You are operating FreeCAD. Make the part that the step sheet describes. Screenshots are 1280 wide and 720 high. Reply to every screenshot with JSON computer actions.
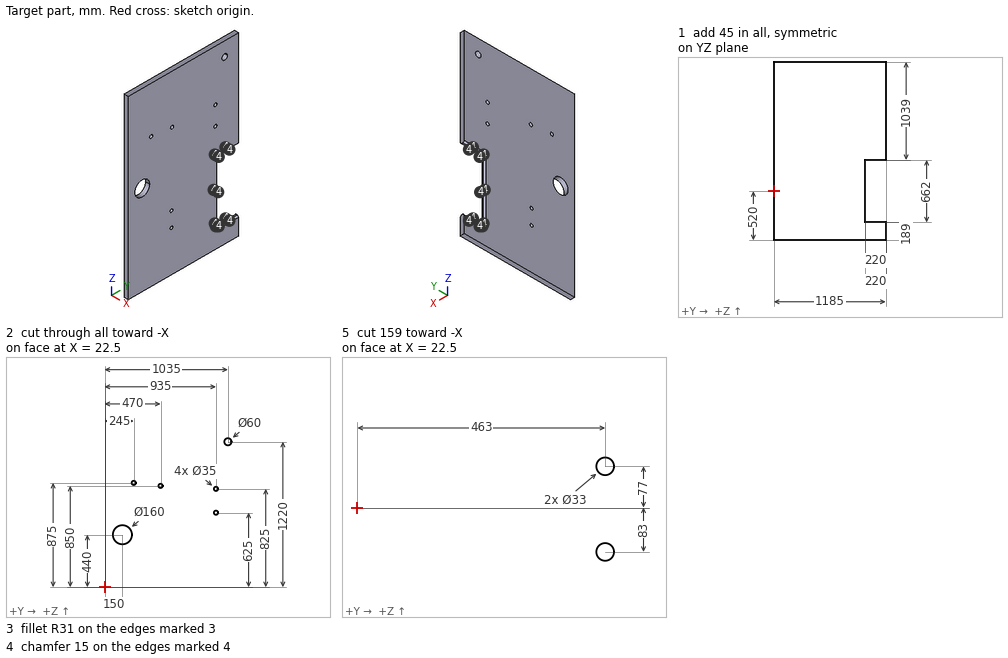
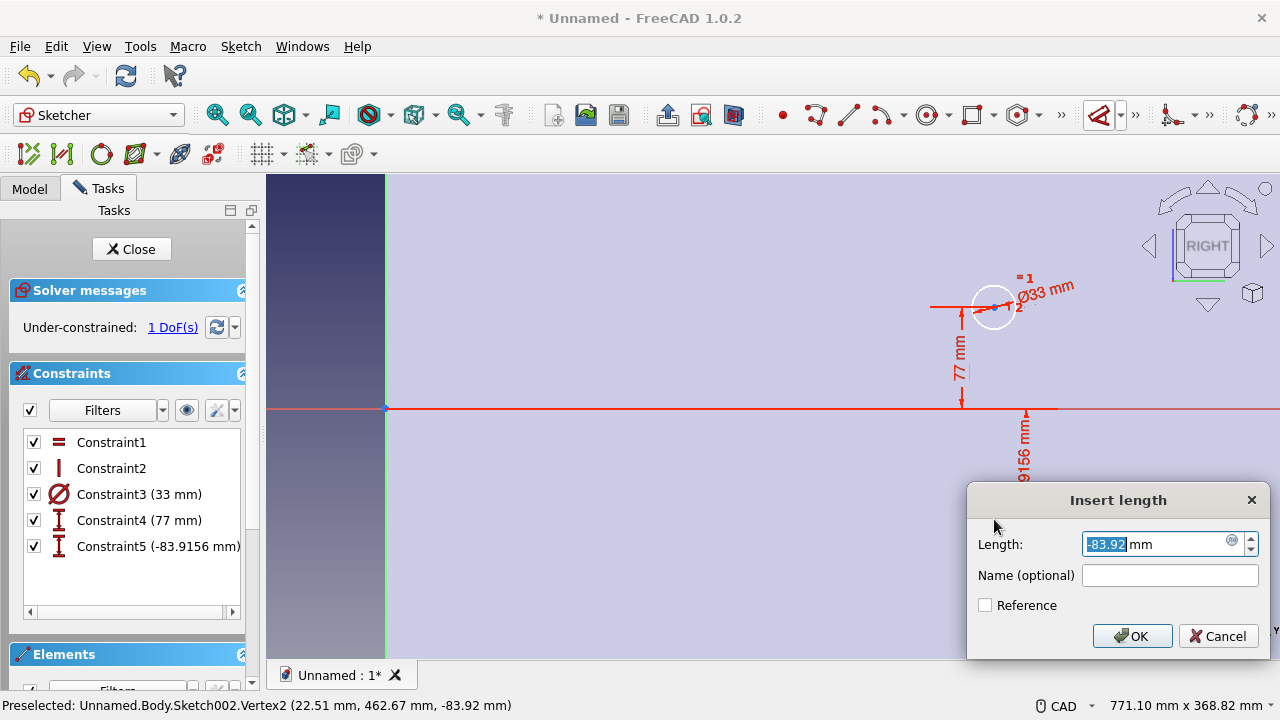
{"action": "type", "text": "-83"}
{"action": "key", "text": "Return"}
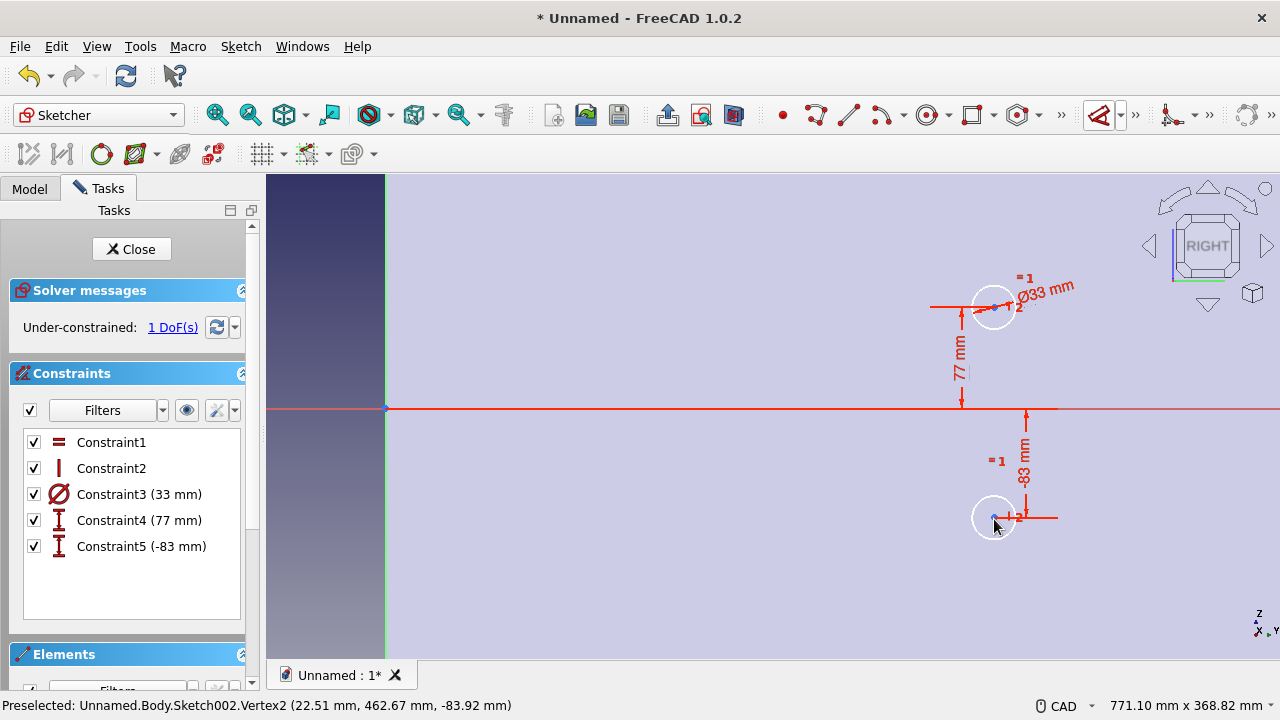
{"action": "left_click", "coordinate": [994, 307]}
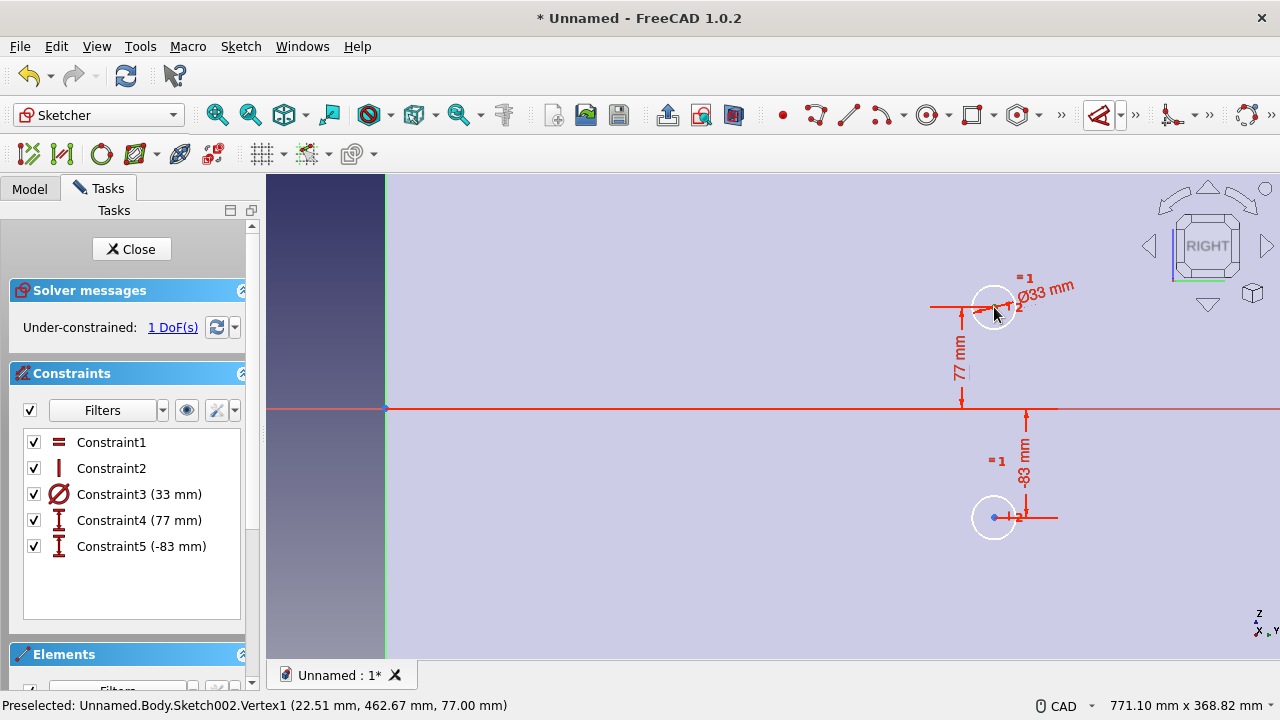
{"action": "left_click", "coordinate": [1120, 116]}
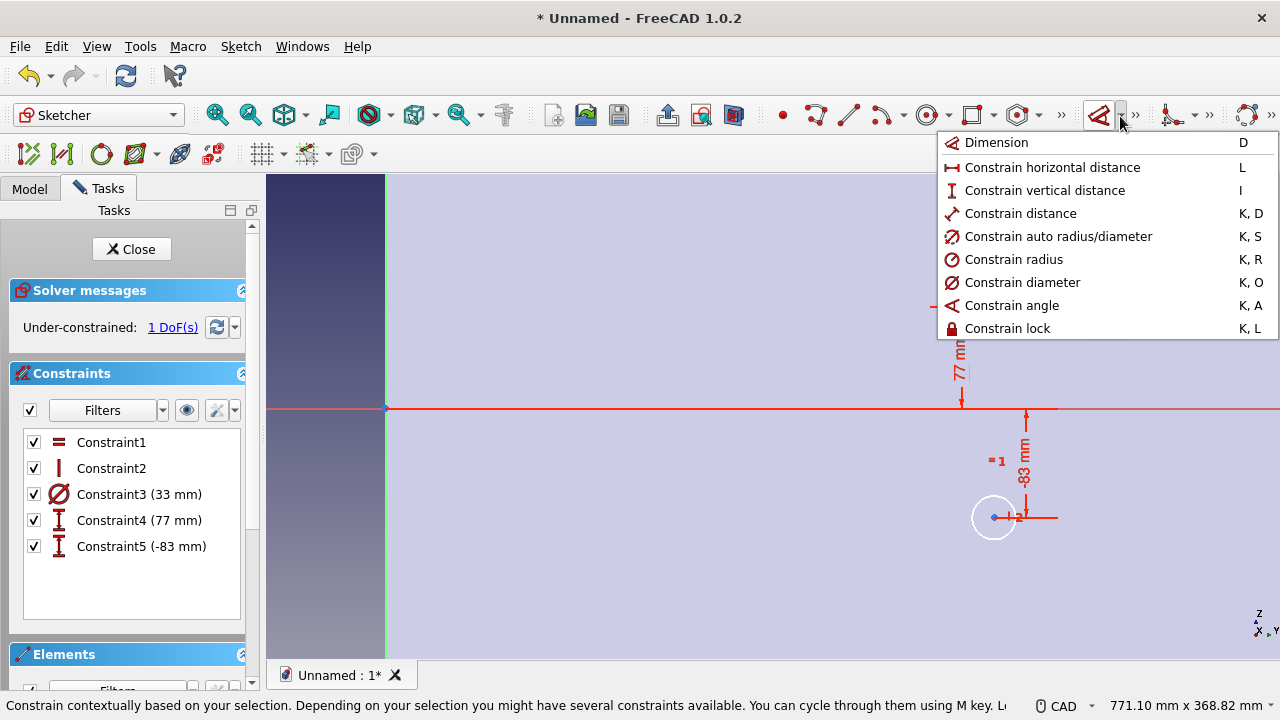
{"action": "left_click", "coordinate": [1108, 168]}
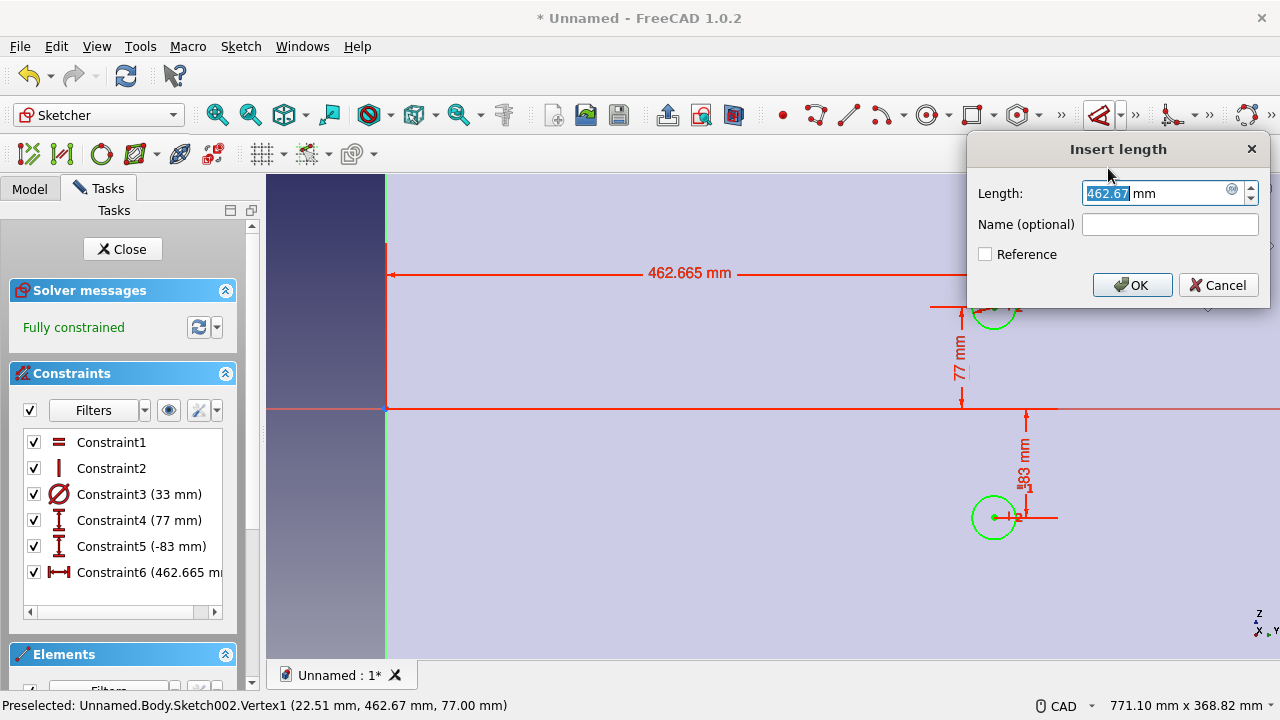
{"action": "type", "text": "463"}
{"action": "key", "text": "Return"}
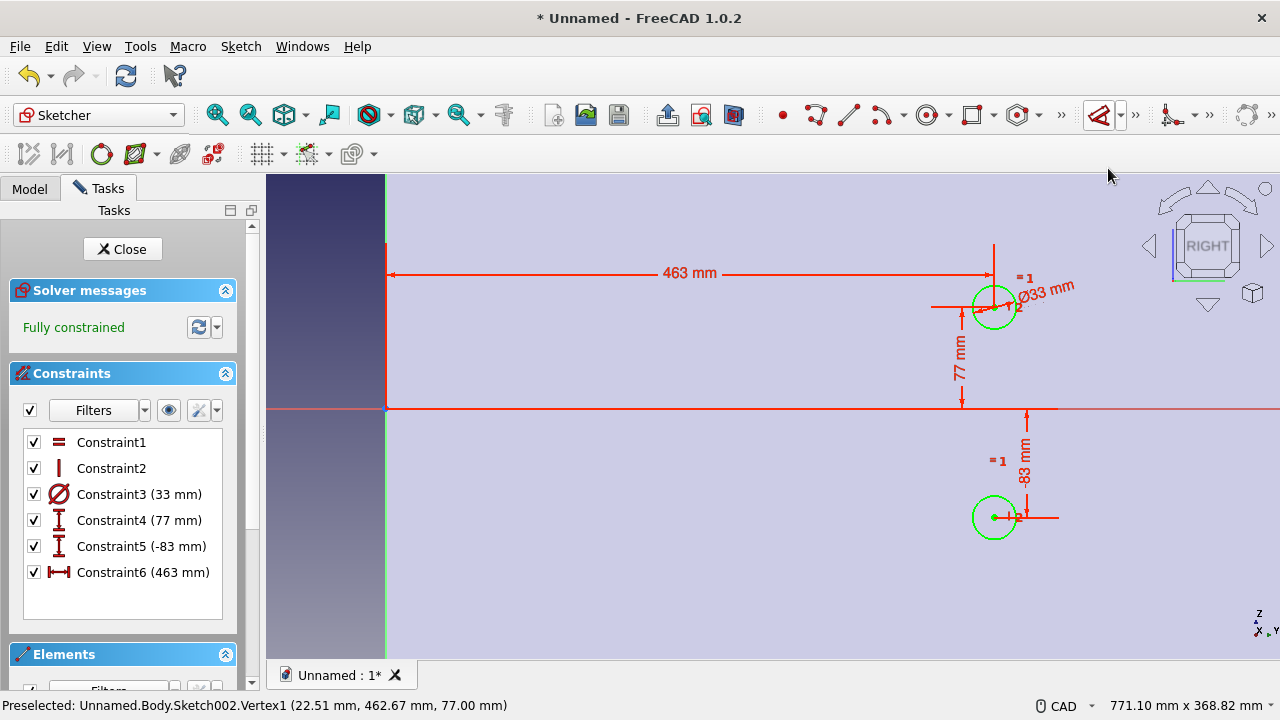
{"action": "left_click", "coordinate": [123, 249]}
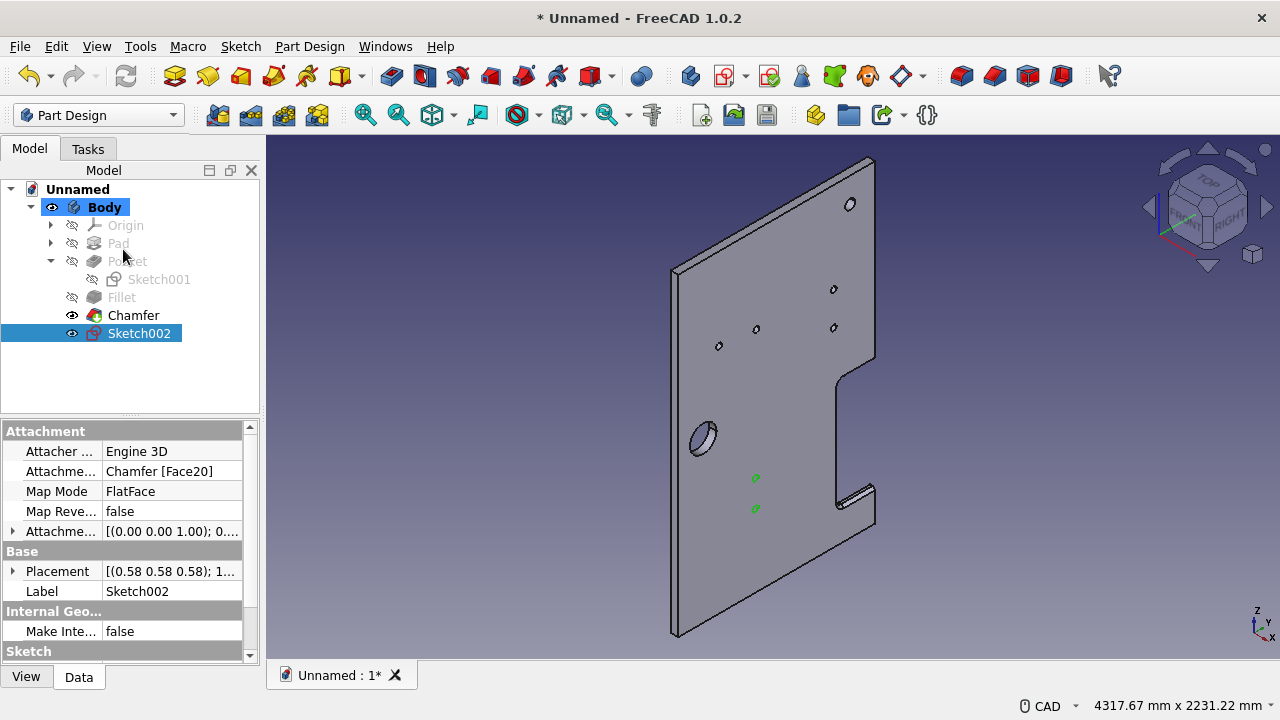
{"action": "left_click", "coordinate": [392, 76]}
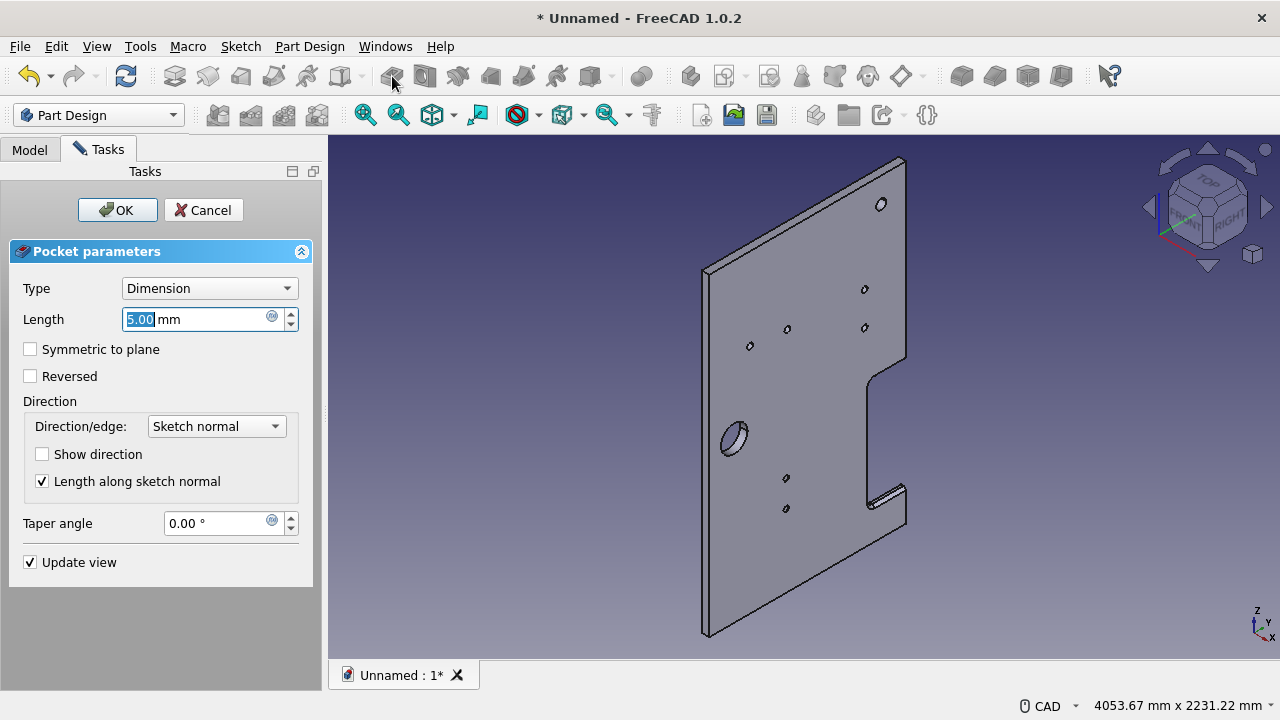
{"action": "type", "text": "159"}
{"action": "key", "text": "Tab"}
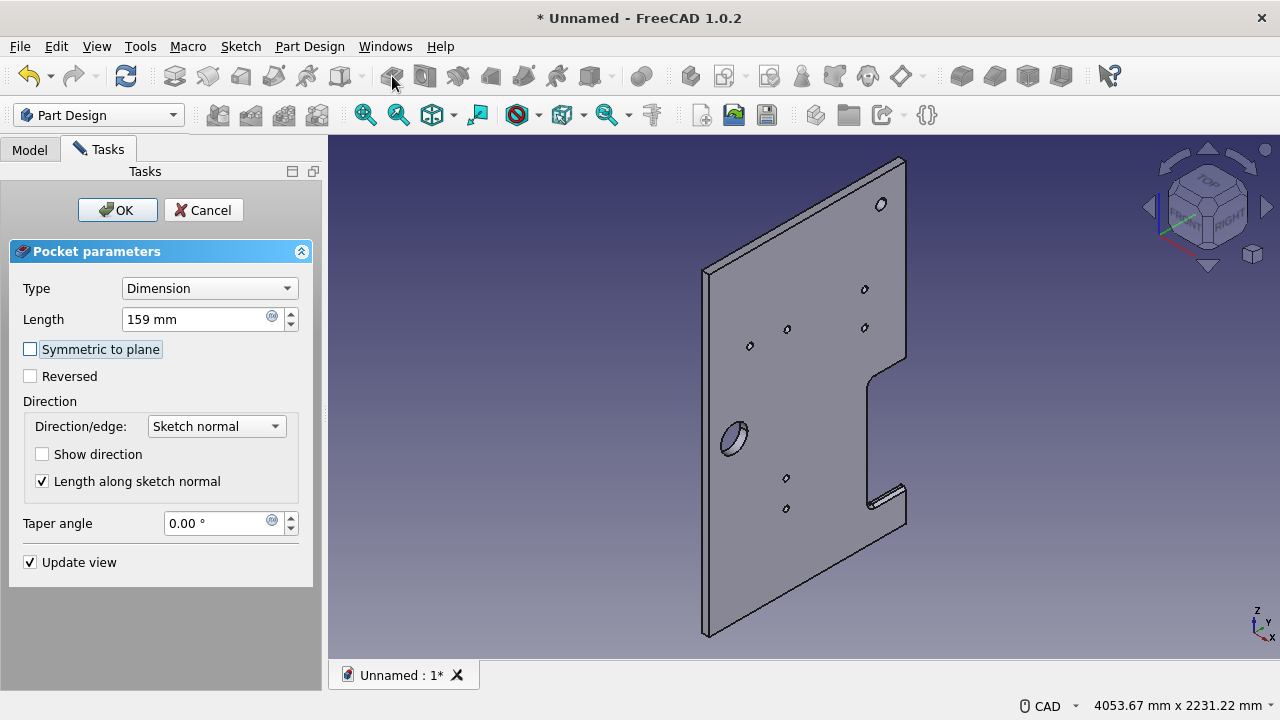
{"action": "left_click", "coordinate": [118, 210]}